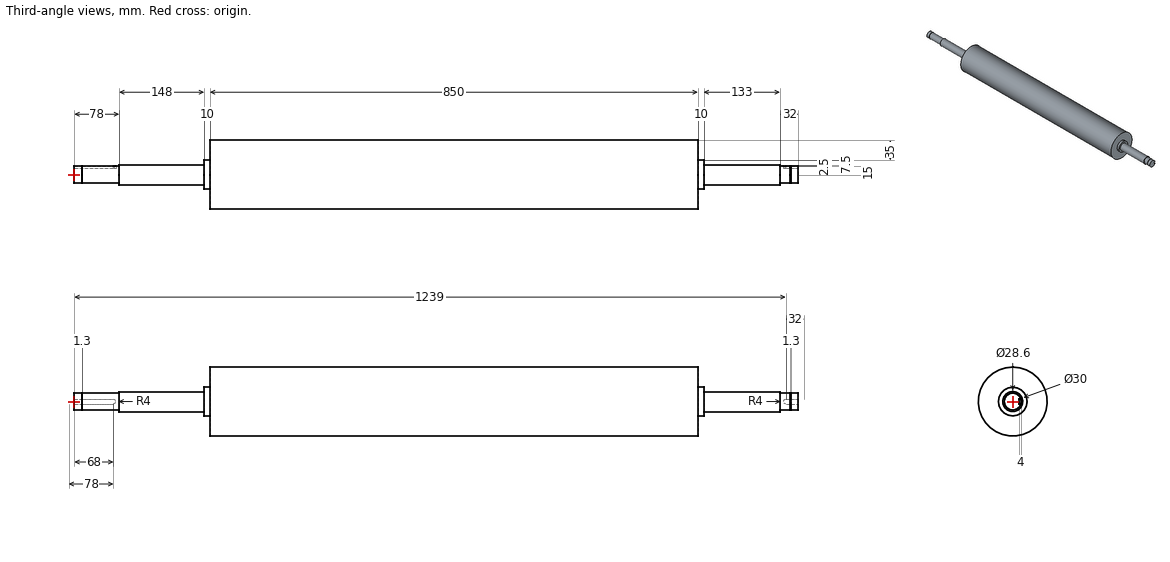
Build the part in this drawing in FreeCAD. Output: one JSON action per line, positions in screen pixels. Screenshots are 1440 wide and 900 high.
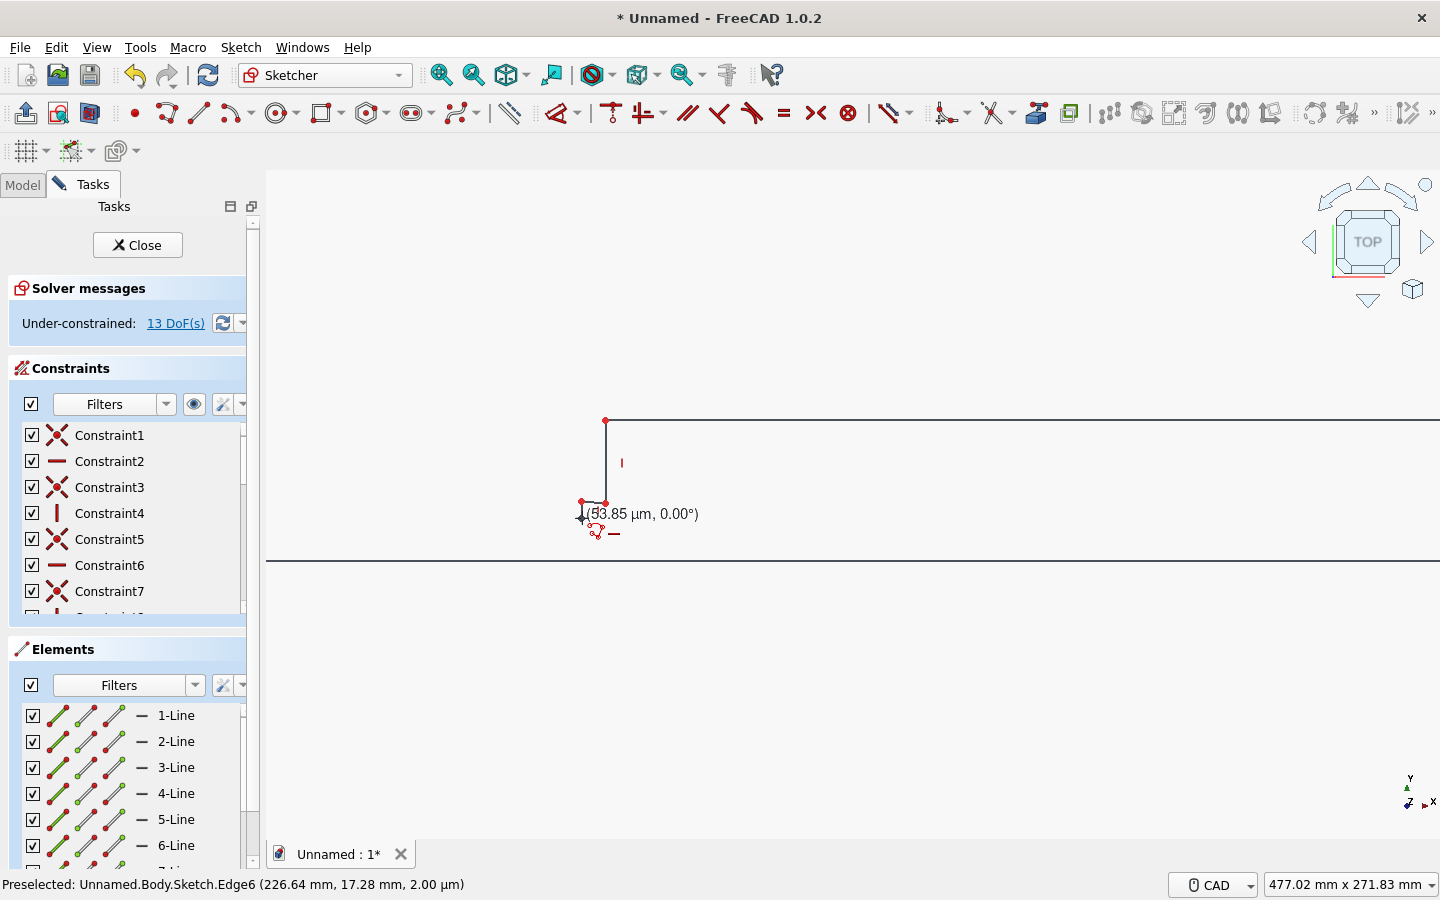
{"action": "scroll", "coordinate": [584, 509], "scroll_direction": "down", "scroll_amount": 8}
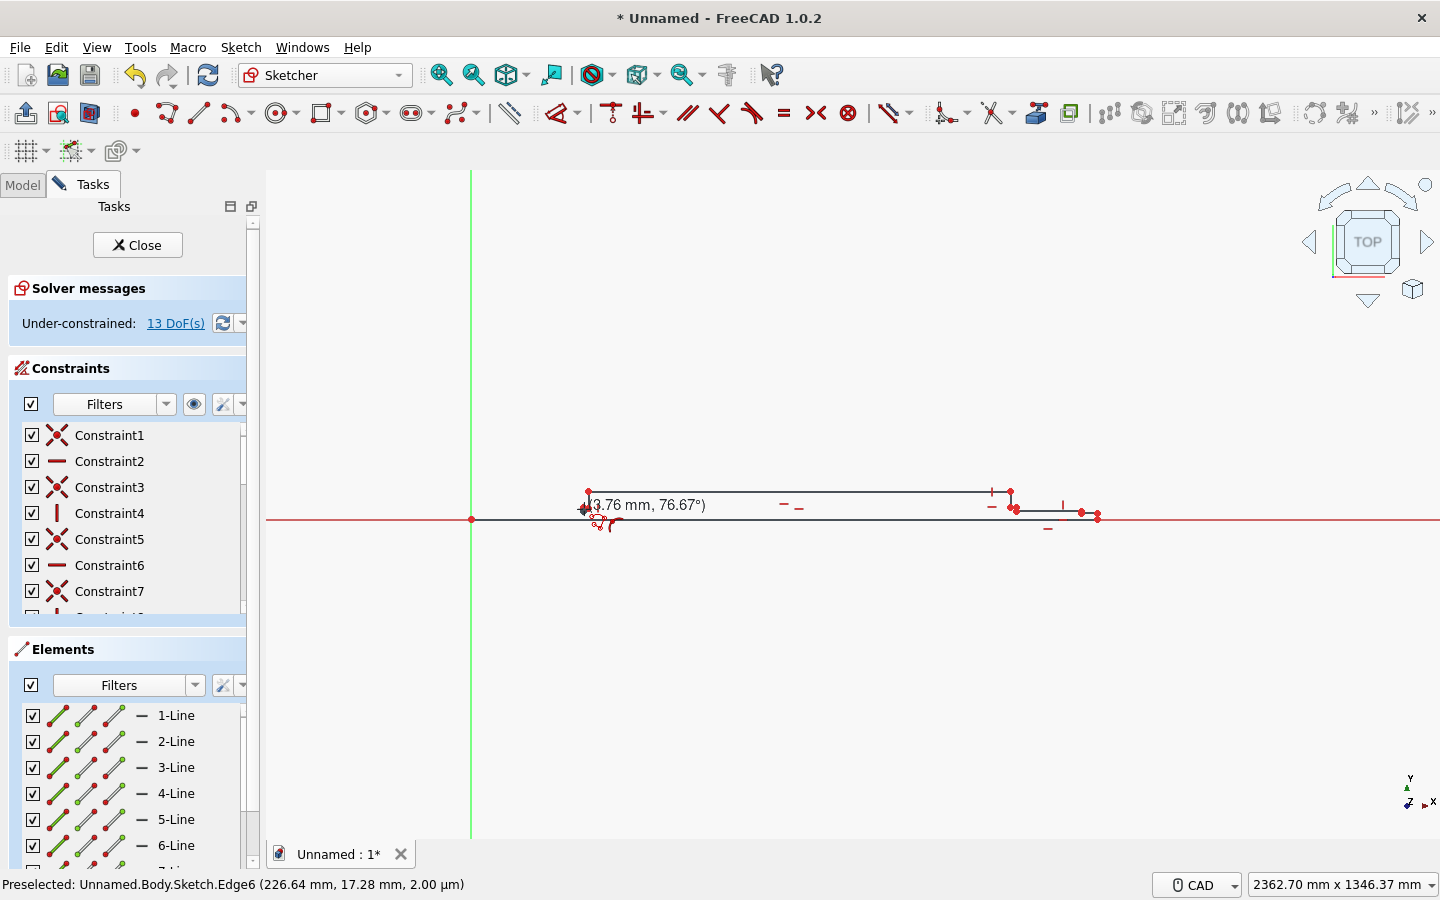
{"action": "scroll", "coordinate": [510, 511], "scroll_direction": "up", "scroll_amount": 4}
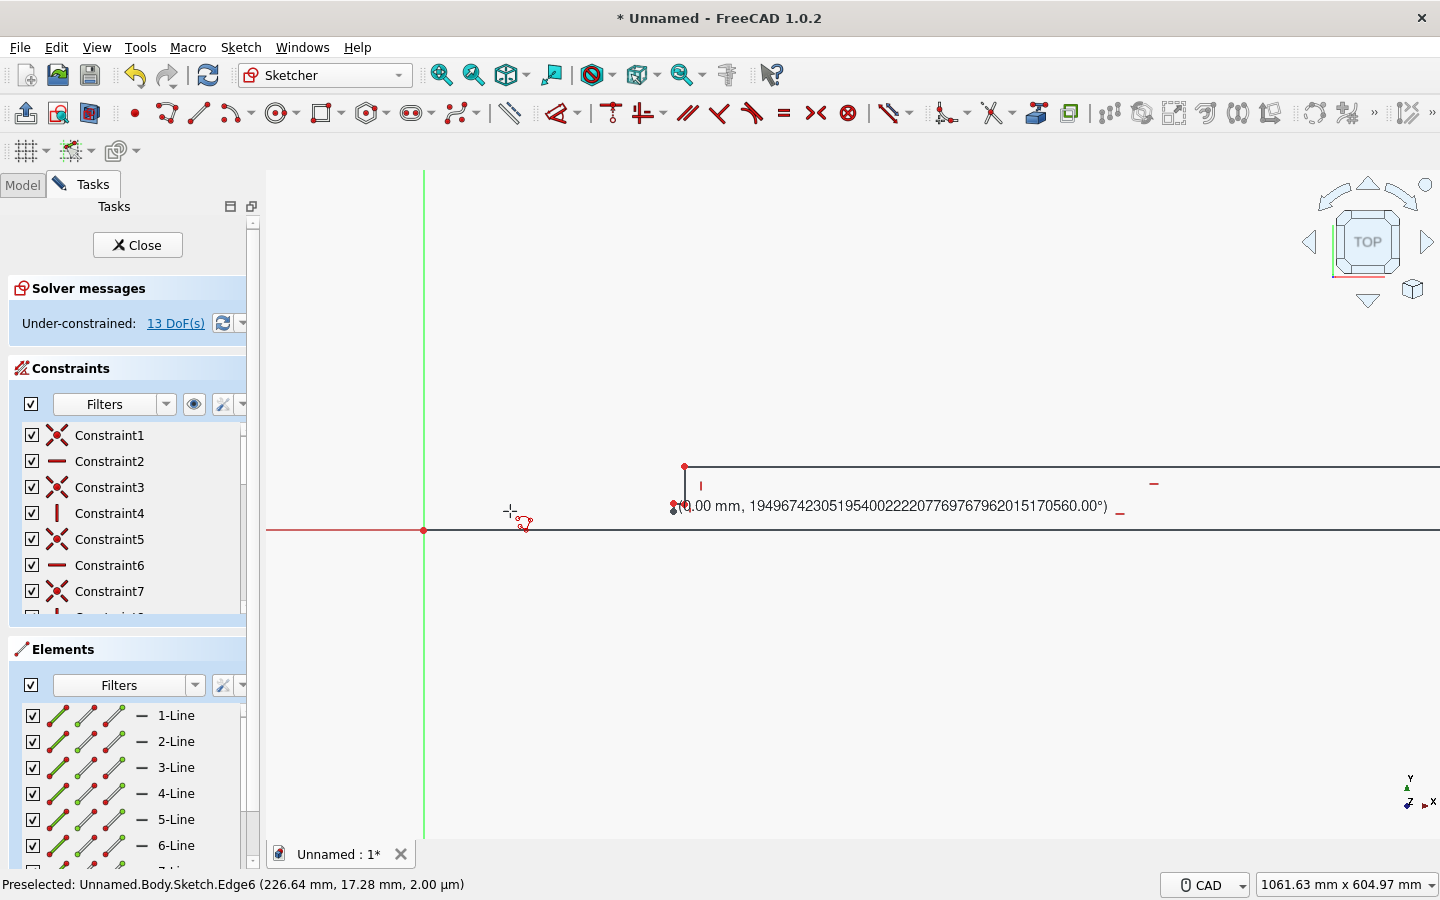
{"action": "left_click", "coordinate": [510, 511]}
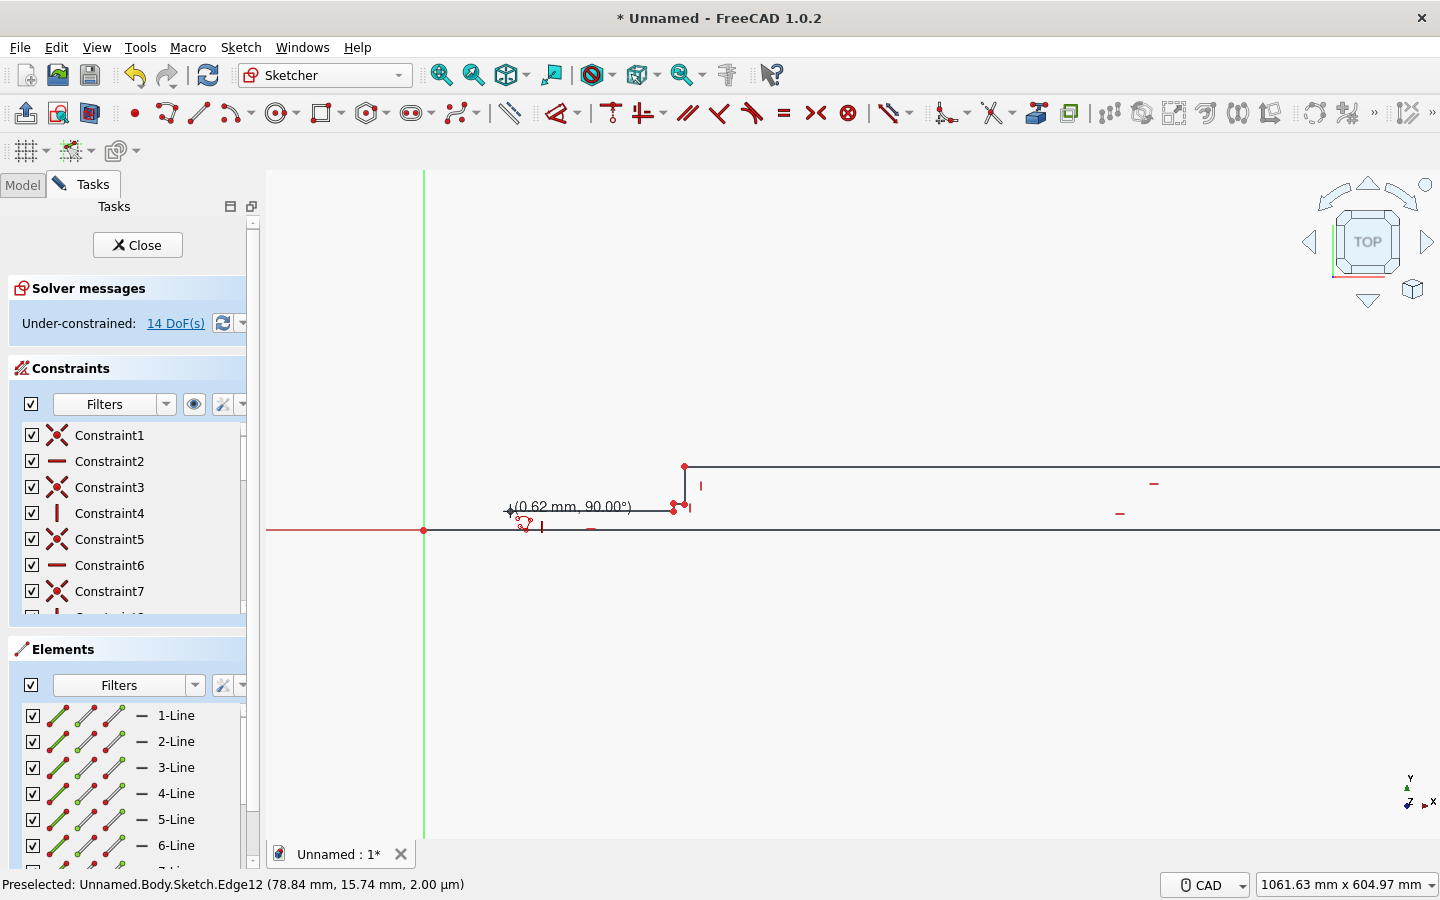
{"action": "scroll", "coordinate": [510, 514], "scroll_direction": "up", "scroll_amount": 9}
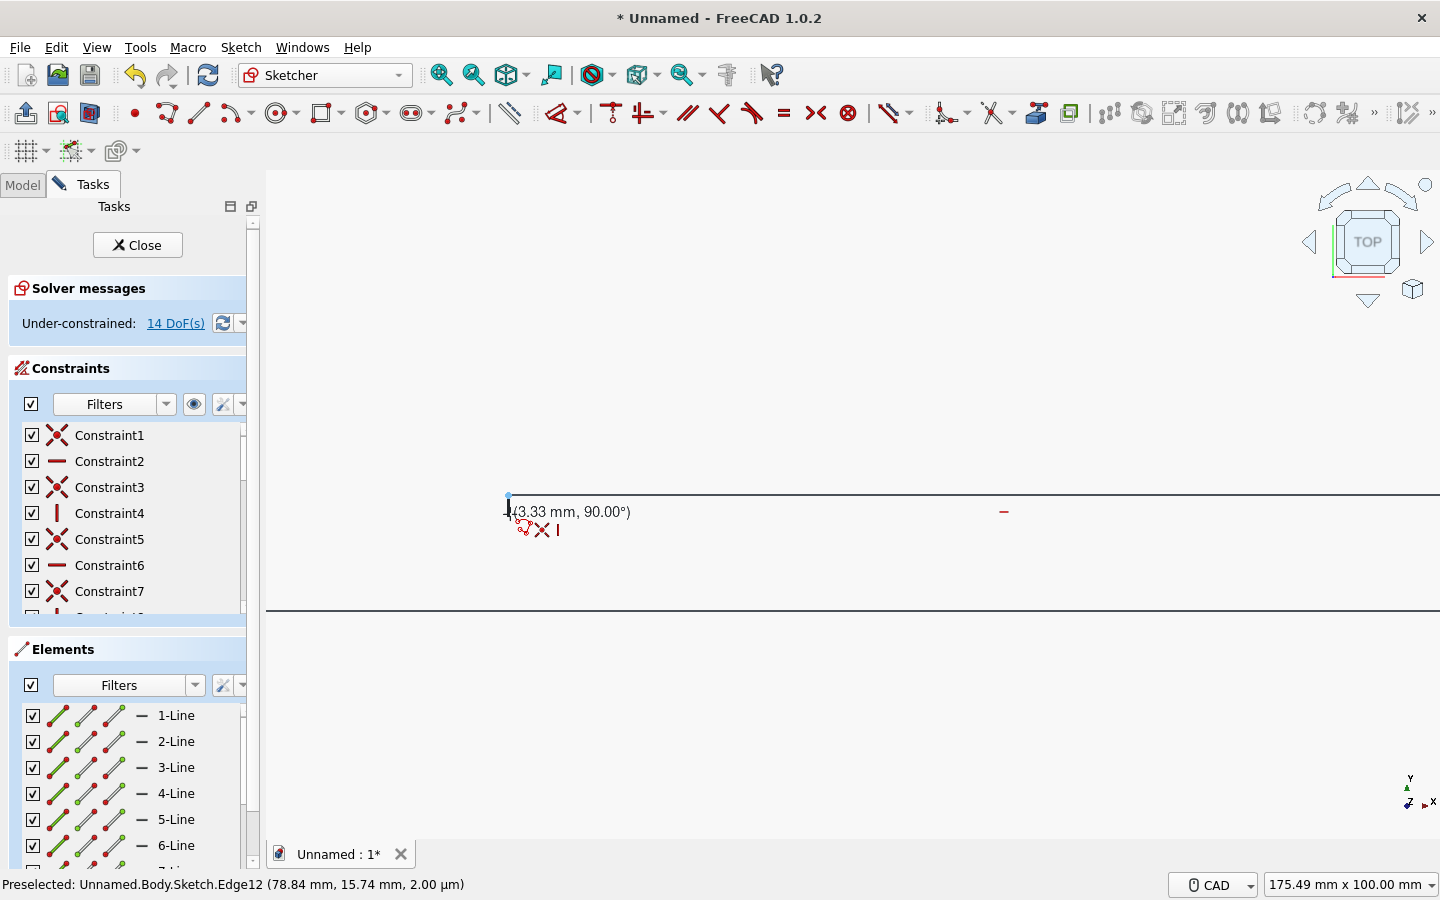
{"action": "left_click", "coordinate": [509, 510]}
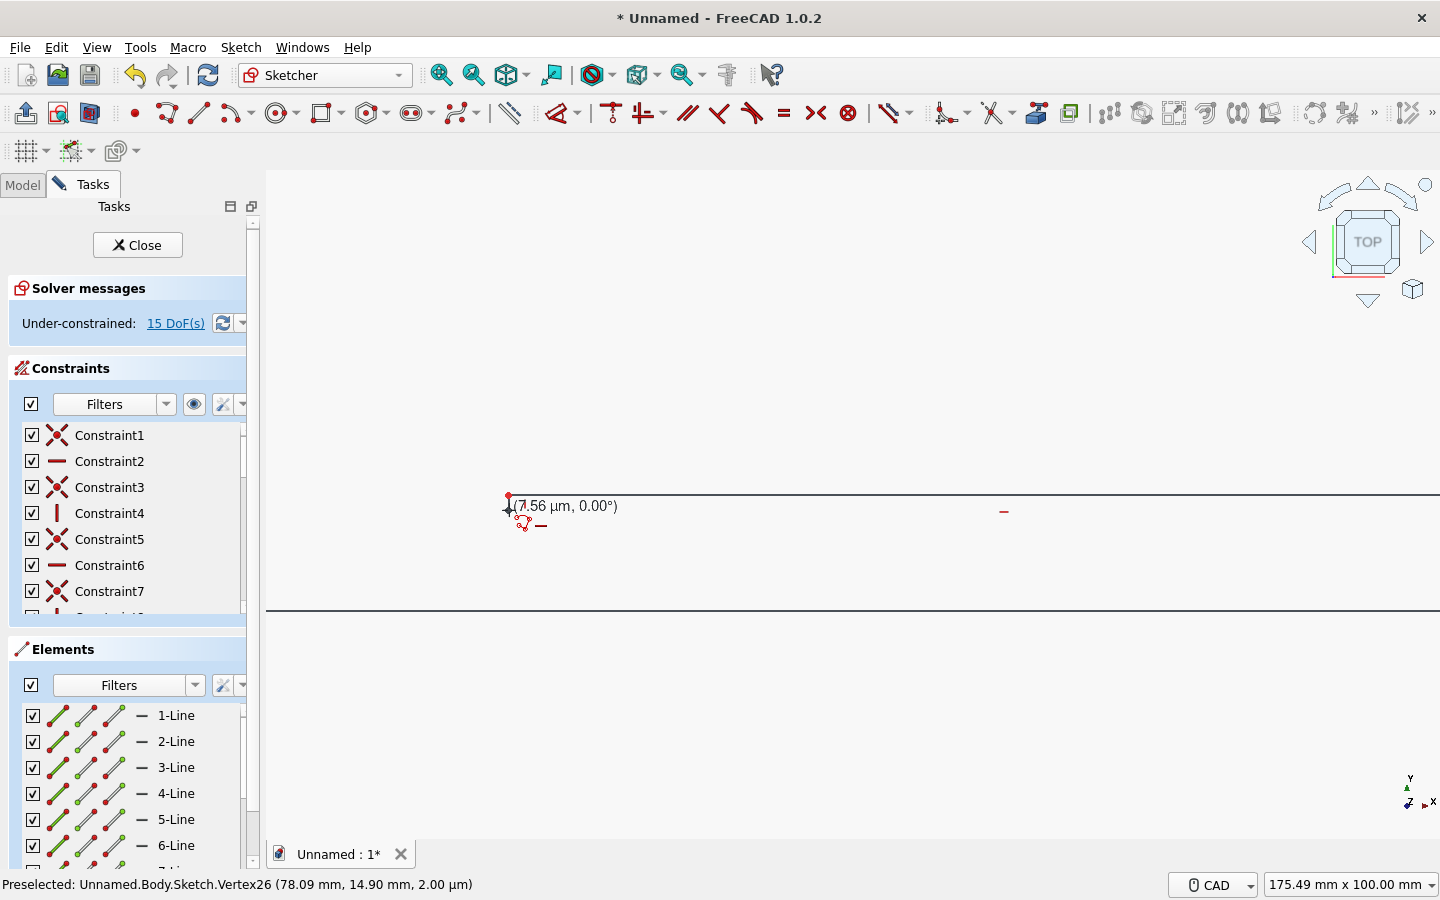
{"action": "scroll", "coordinate": [510, 512], "scroll_direction": "down", "scroll_amount": 13}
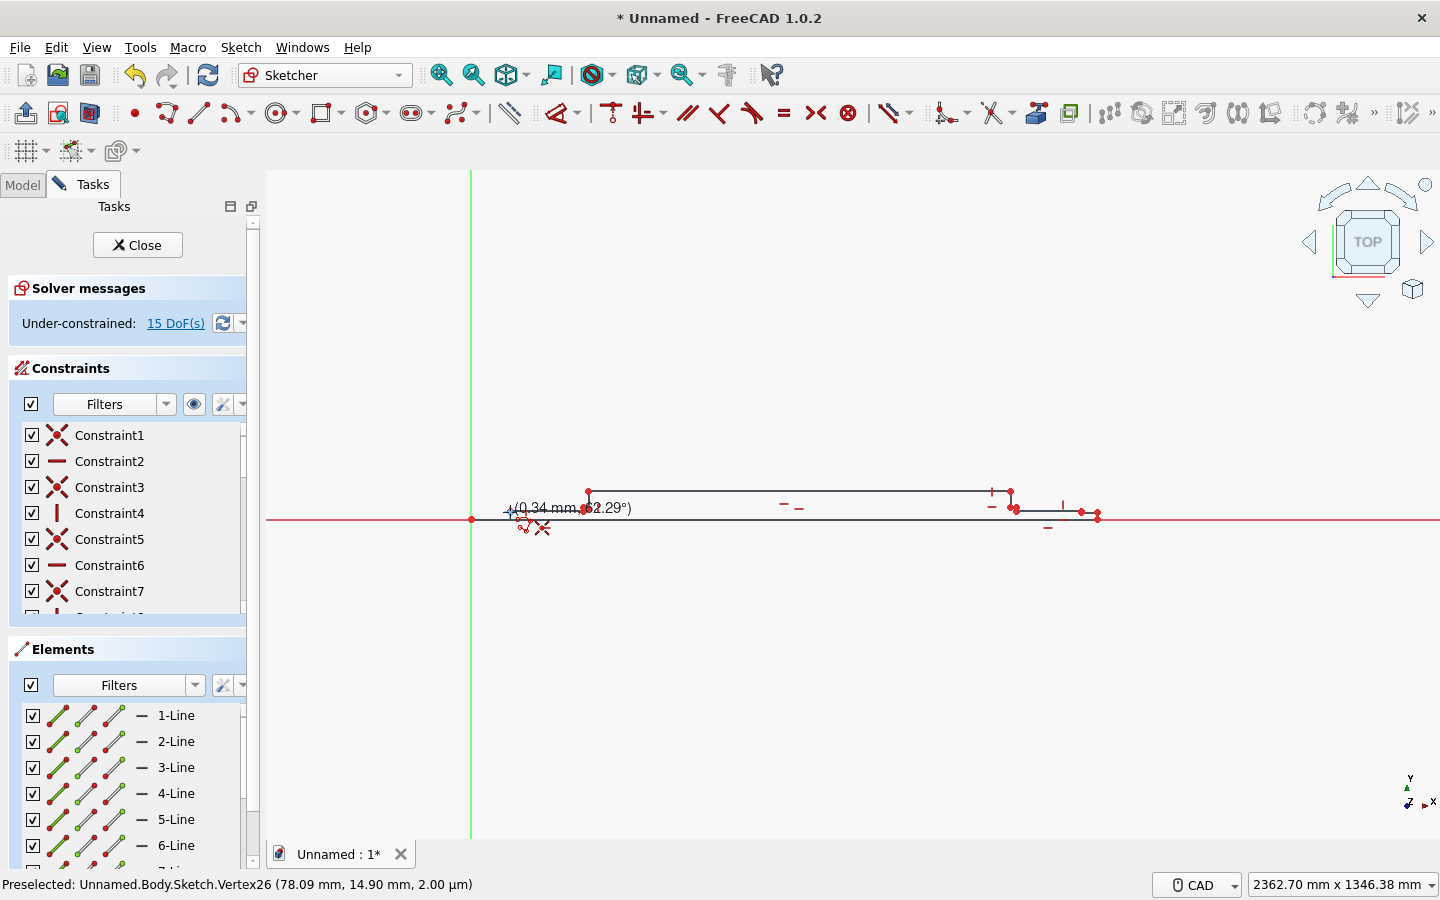
{"action": "scroll", "coordinate": [471, 512], "scroll_direction": "up", "scroll_amount": 4}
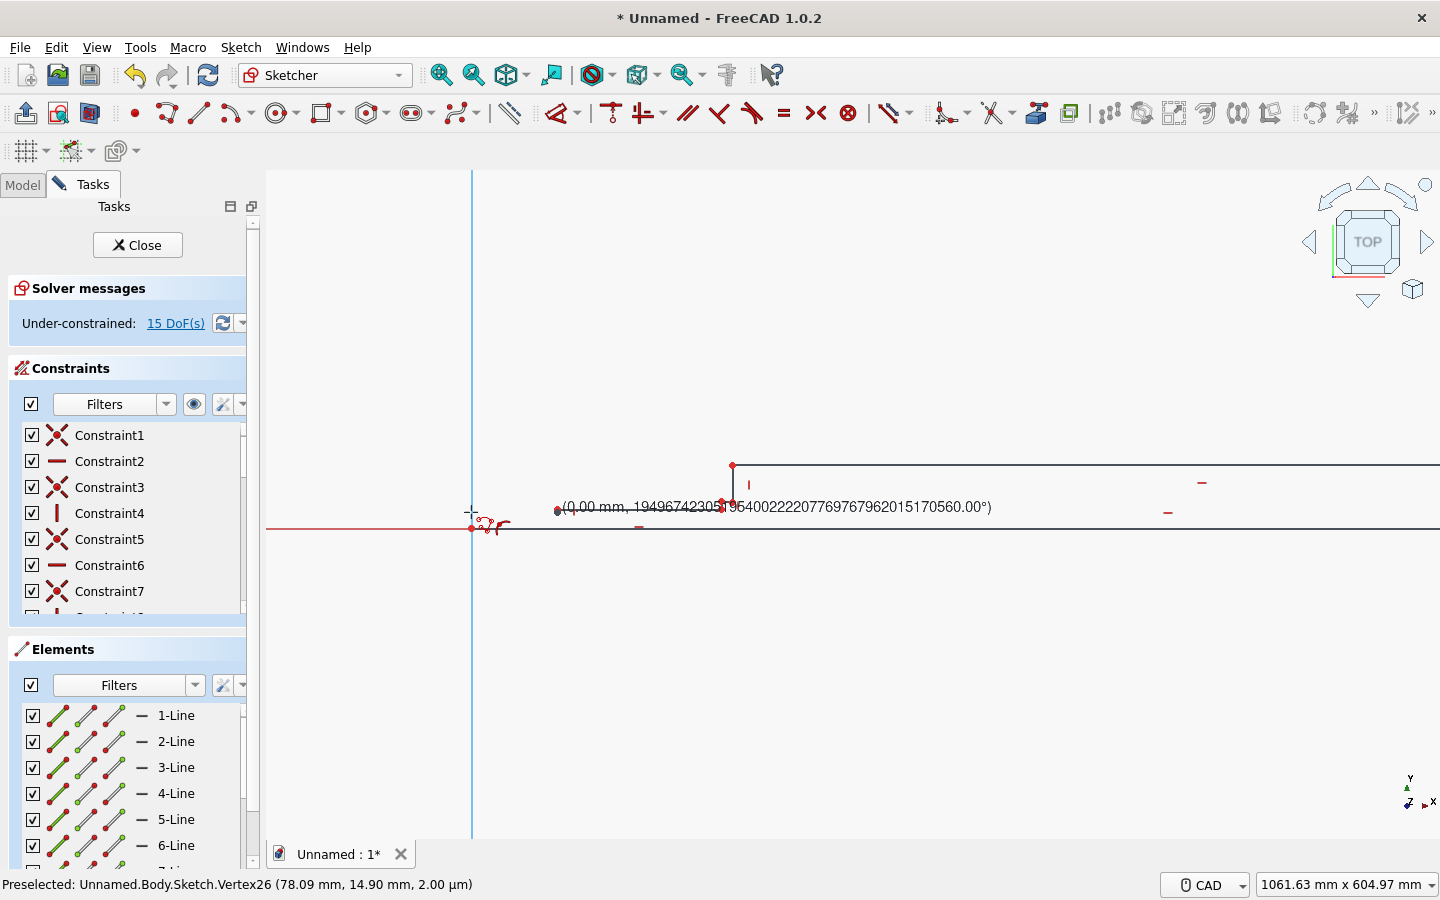
{"action": "left_click", "coordinate": [481, 512]}
{"action": "left_click", "coordinate": [472, 529]}
{"action": "key", "text": "Escape"}
{"action": "key", "text": "Escape"}